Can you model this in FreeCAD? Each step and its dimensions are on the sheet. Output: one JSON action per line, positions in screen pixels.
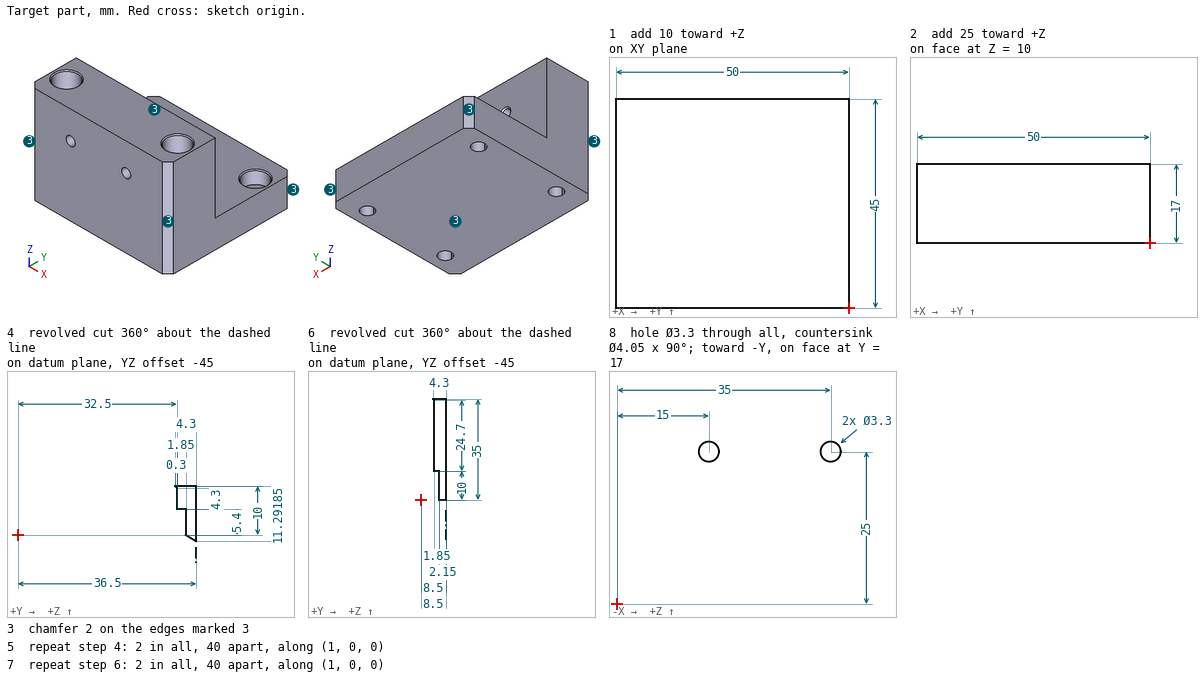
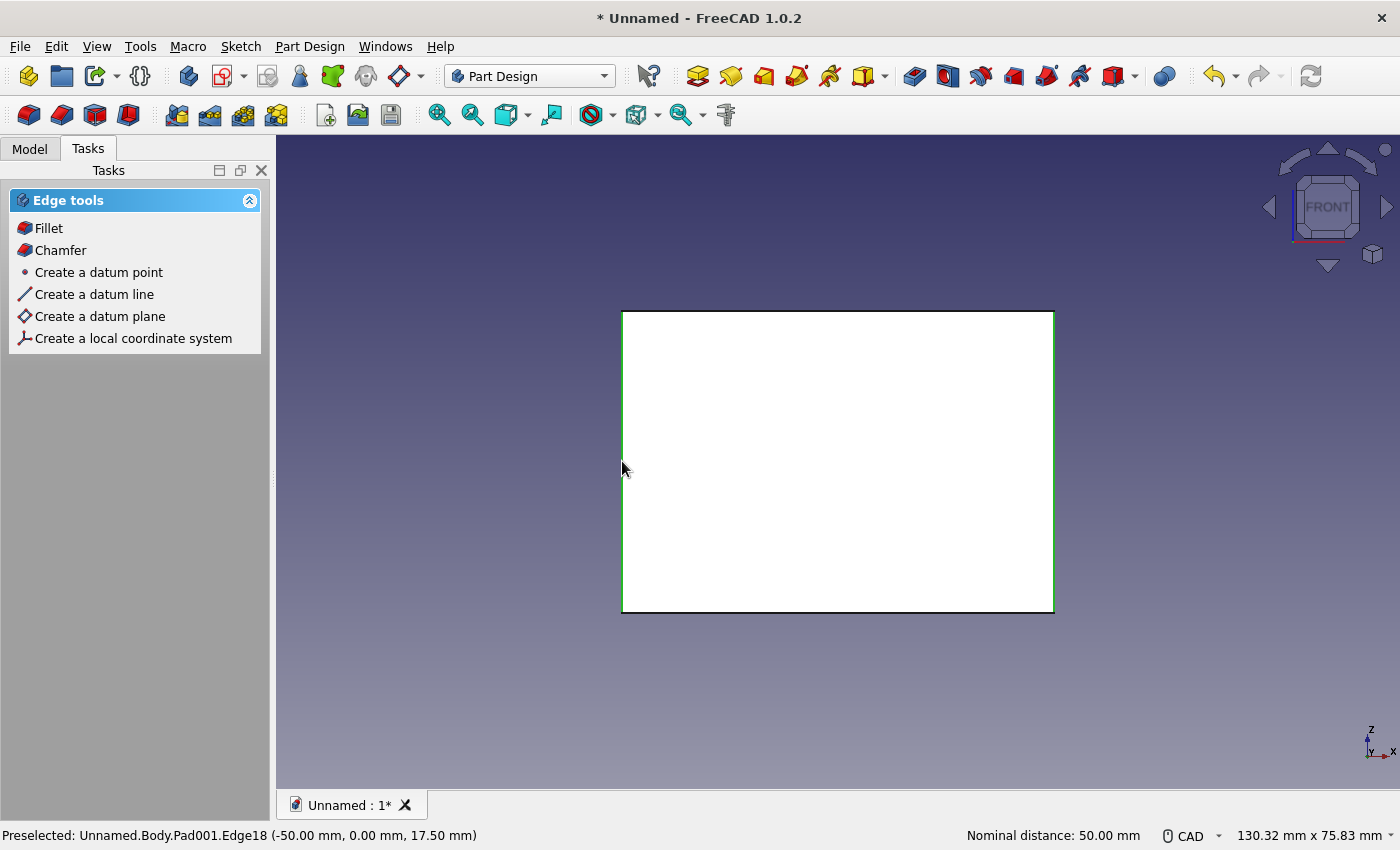
{"action": "key", "text": "3"}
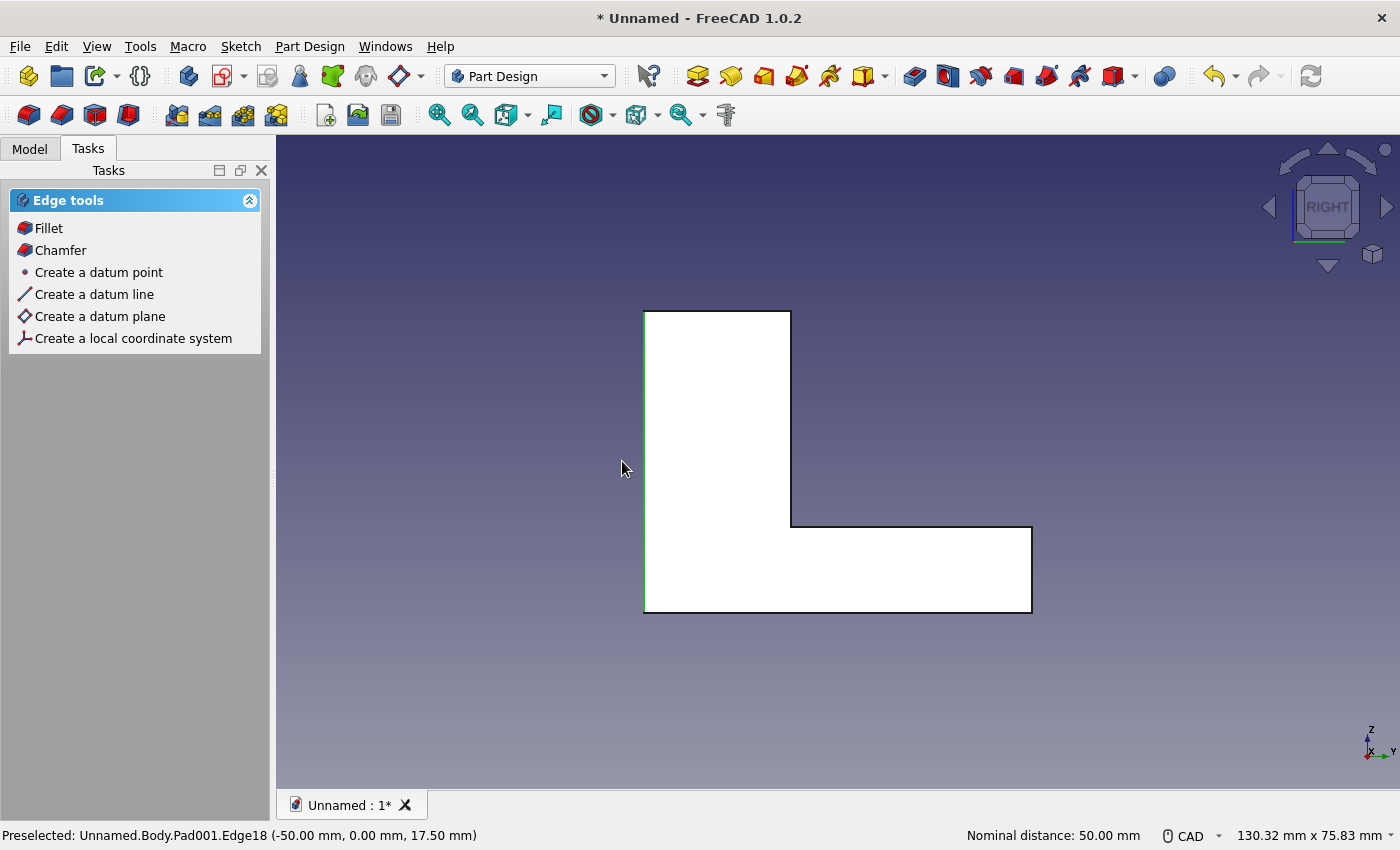
{"action": "left_click", "coordinate": [1032, 569], "text": "ctrl"}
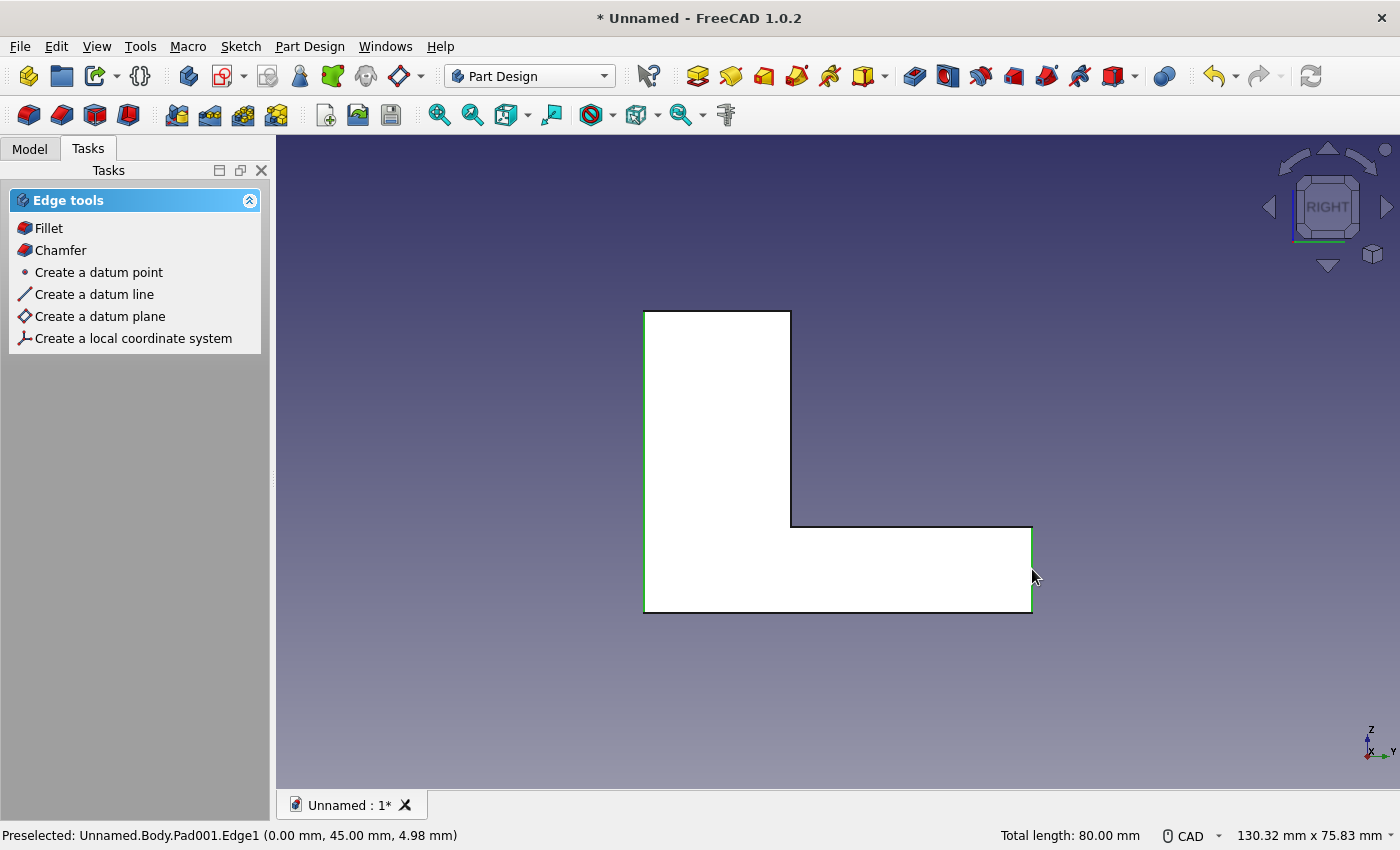
{"action": "key", "text": "5"}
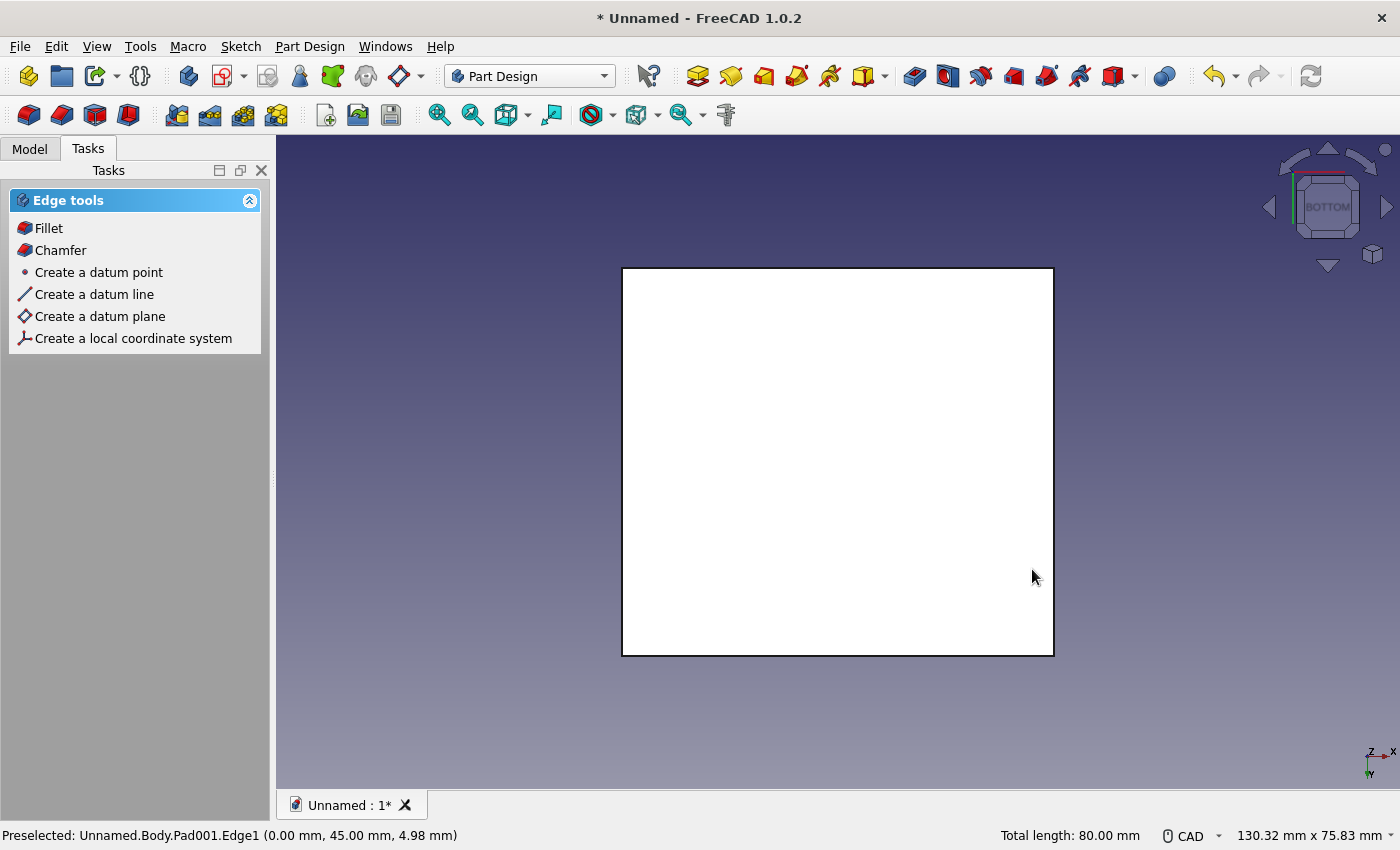
{"action": "key", "text": "4"}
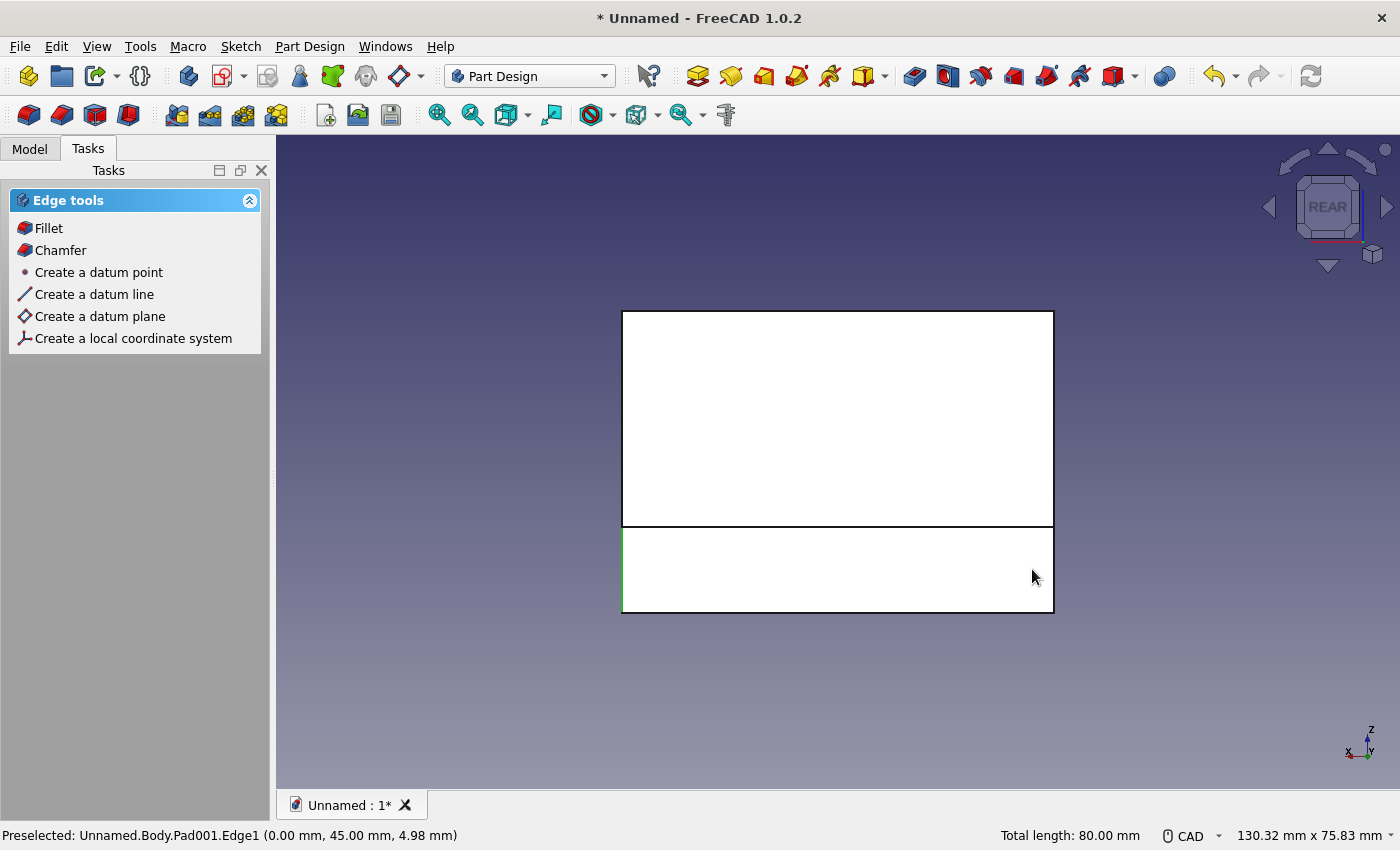
{"action": "left_click", "coordinate": [1054, 569], "text": "ctrl"}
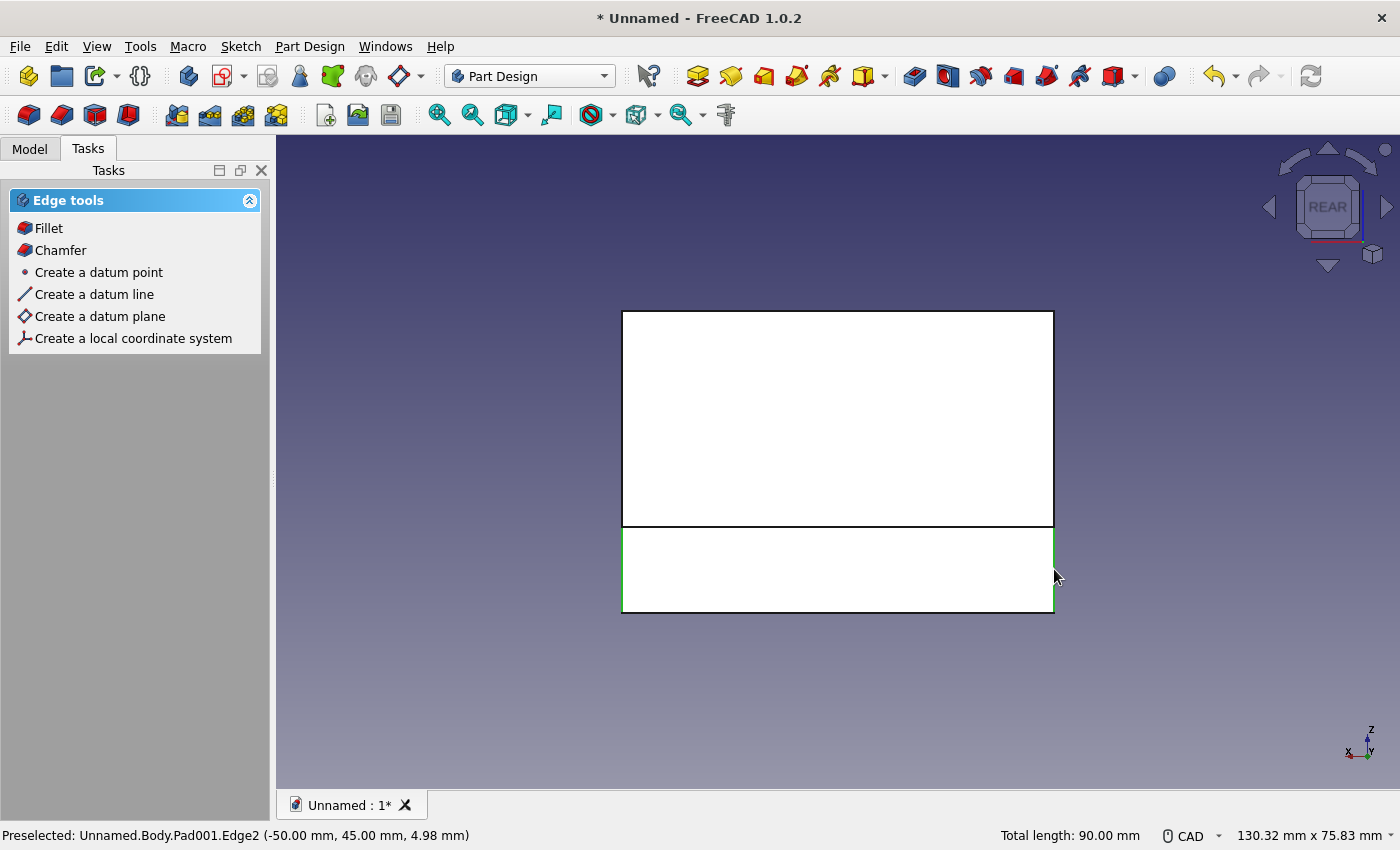
{"action": "left_click", "coordinate": [62, 116]}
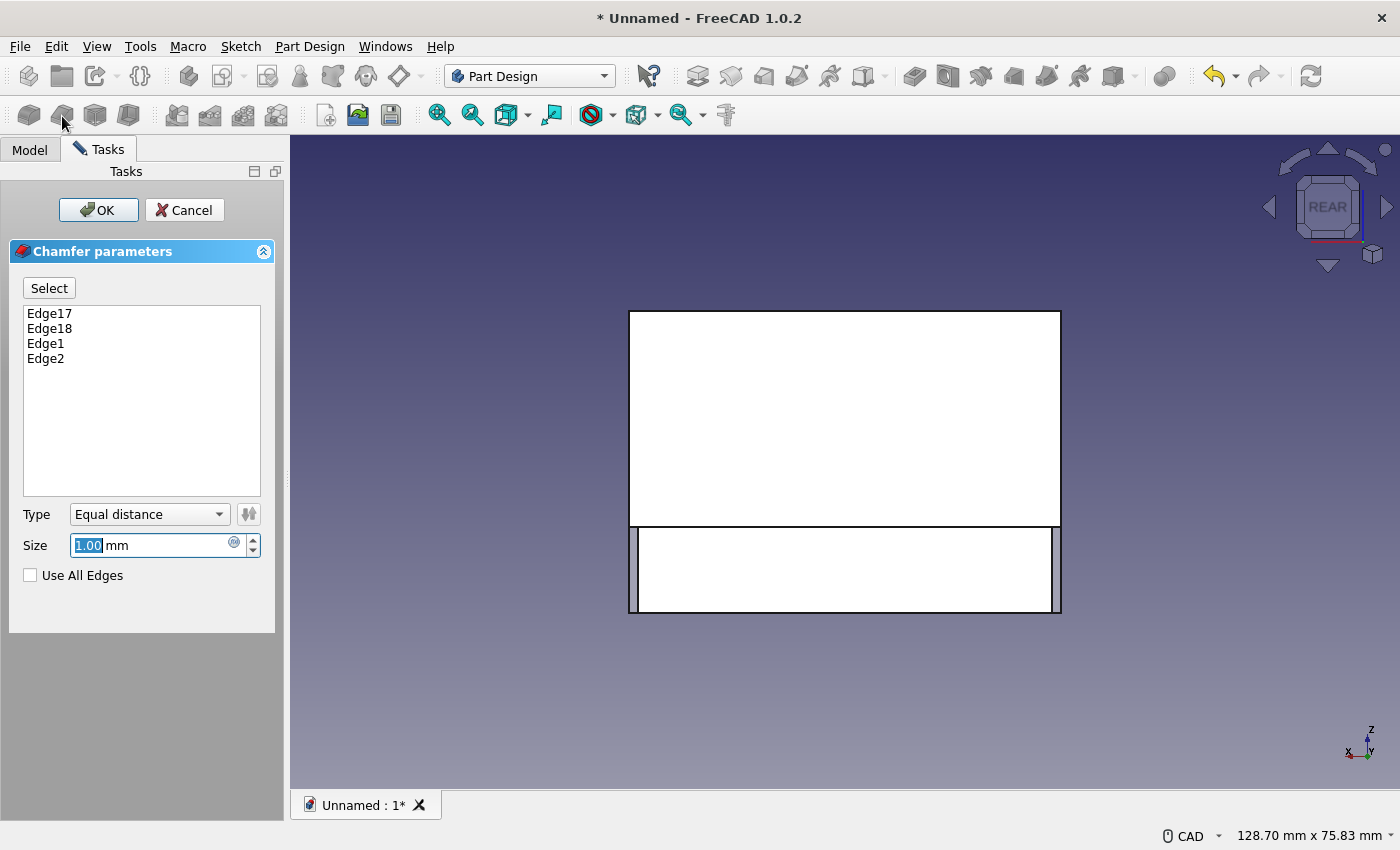
{"action": "type", "text": "2"}
{"action": "key", "text": "Tab"}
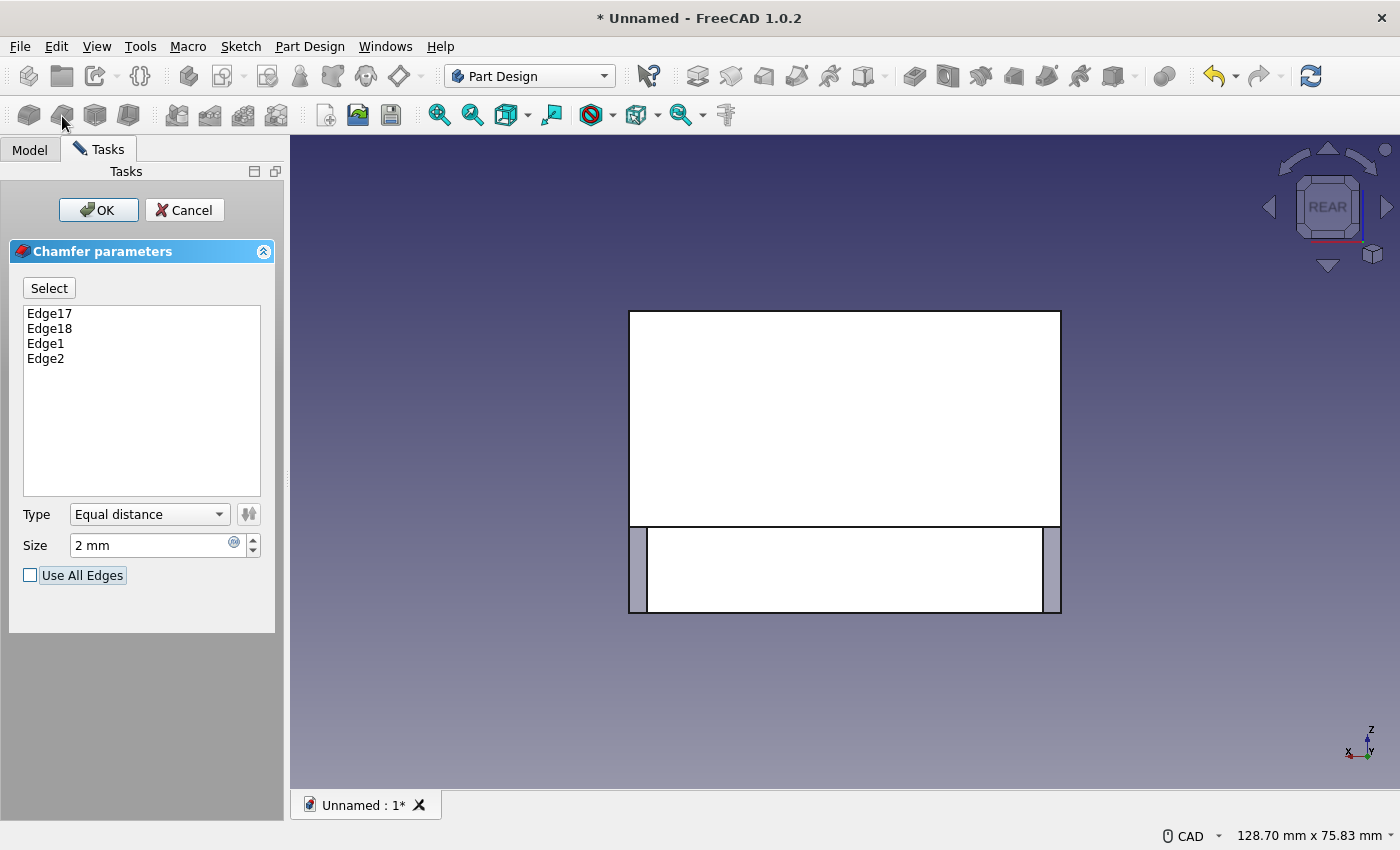
{"action": "left_click", "coordinate": [99, 210]}